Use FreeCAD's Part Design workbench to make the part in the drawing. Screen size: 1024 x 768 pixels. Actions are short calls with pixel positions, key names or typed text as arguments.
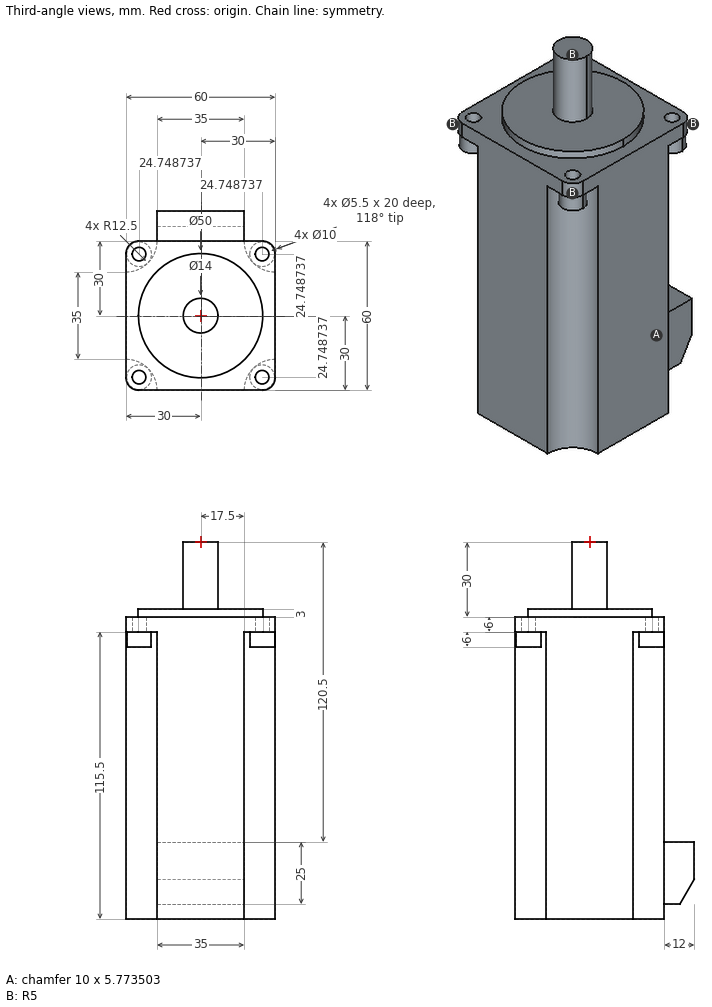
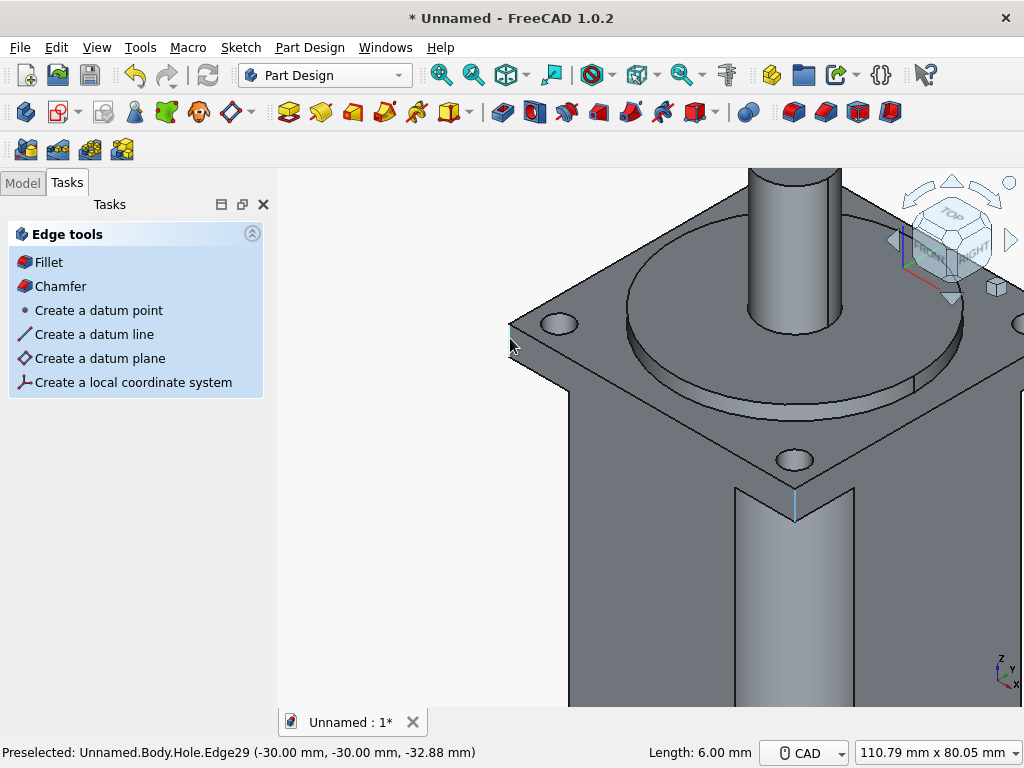
click(442, 76)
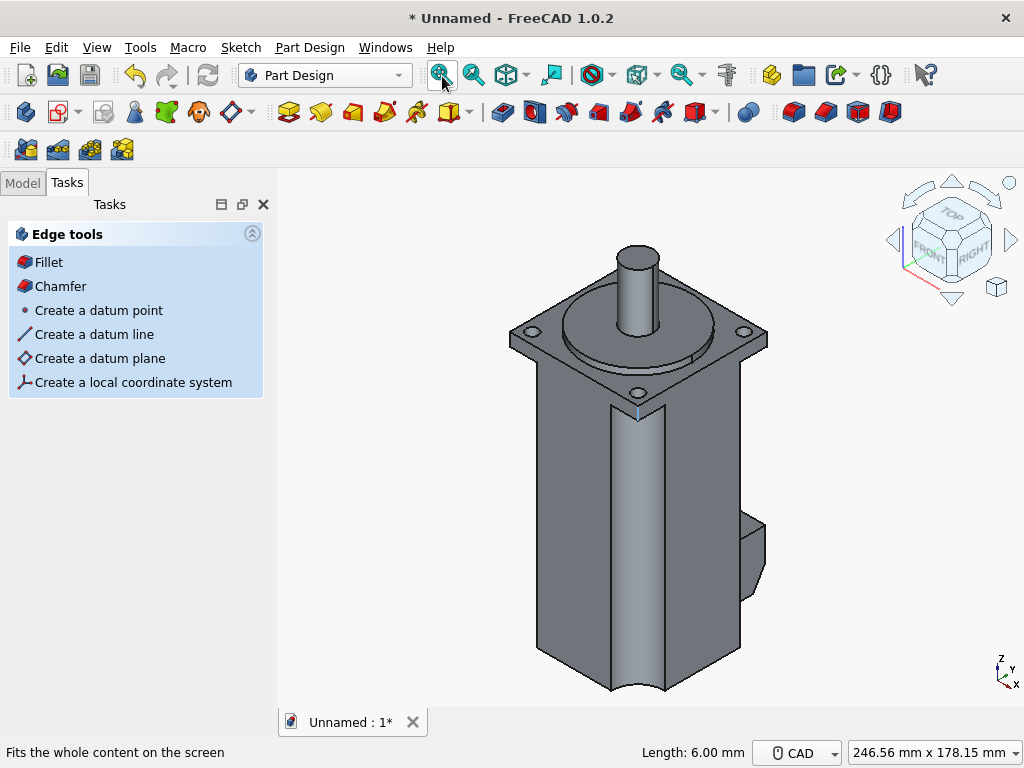
key(2)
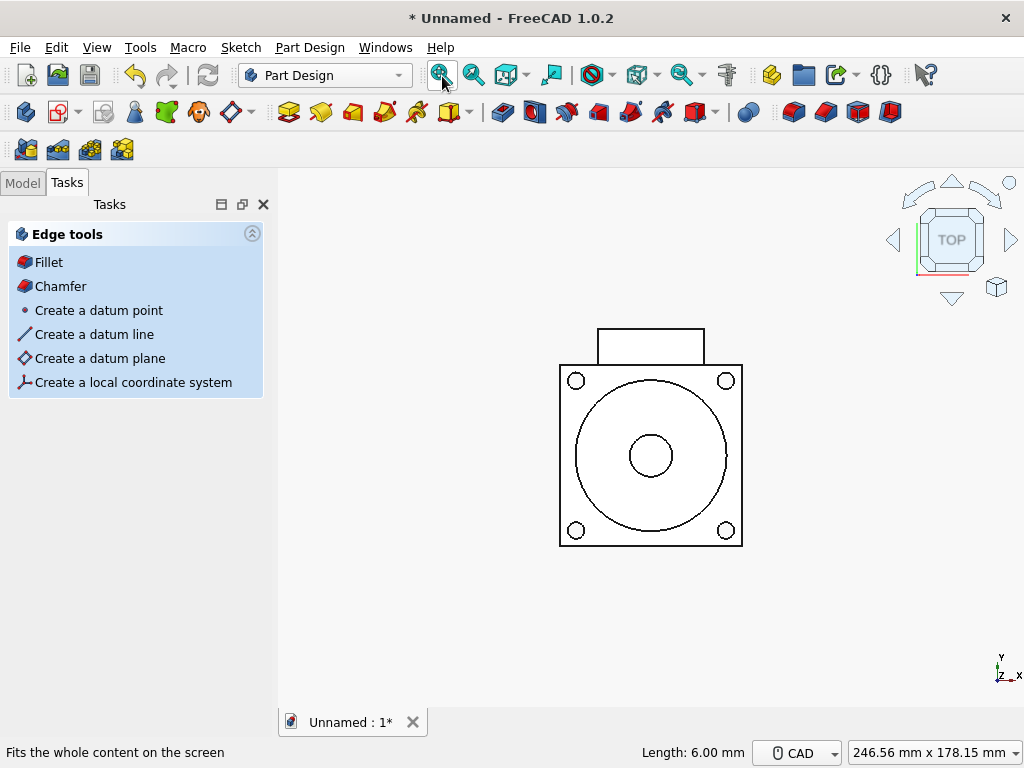
click(442, 76)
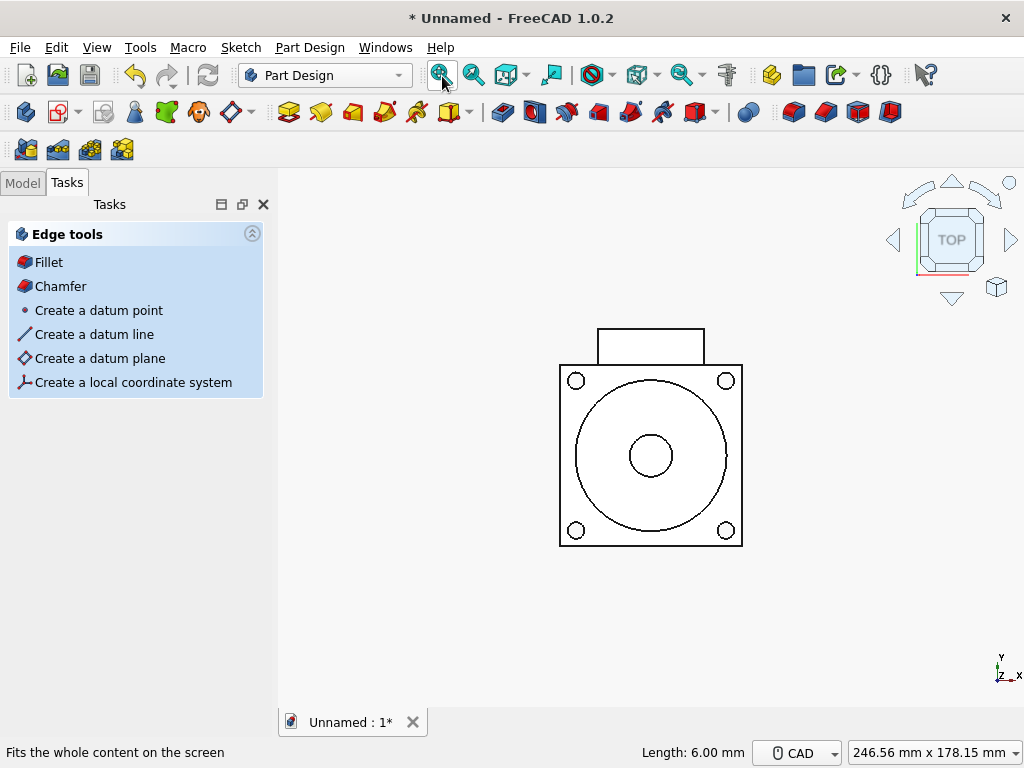
scroll(560, 545, up, 4)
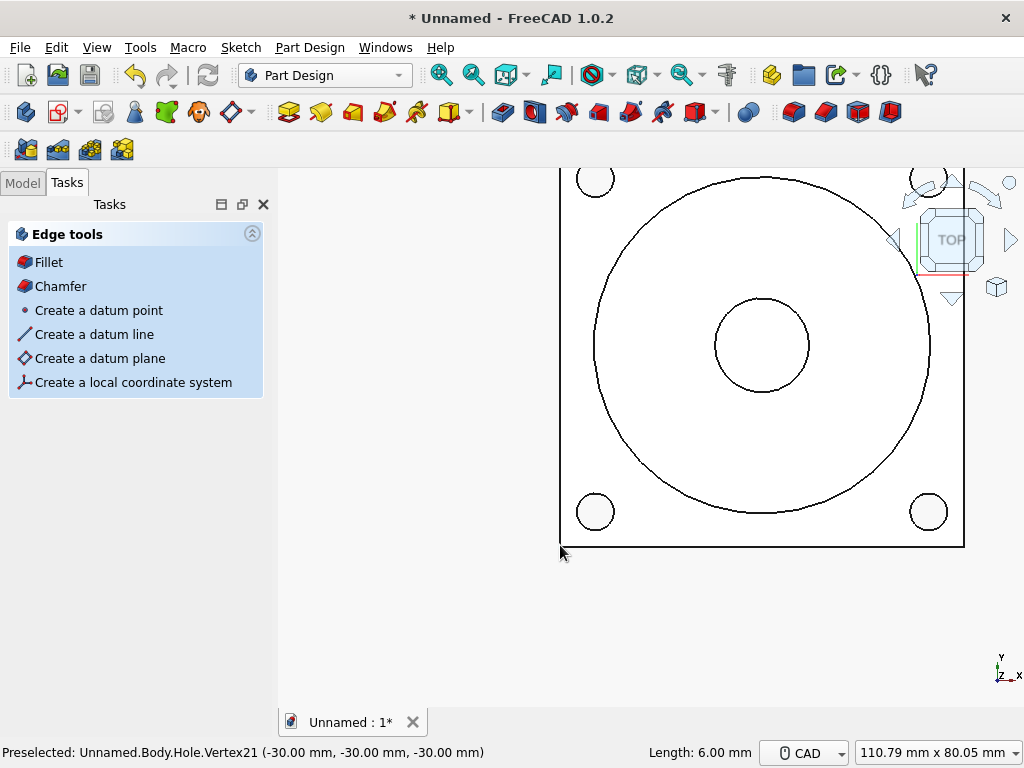
click(442, 76)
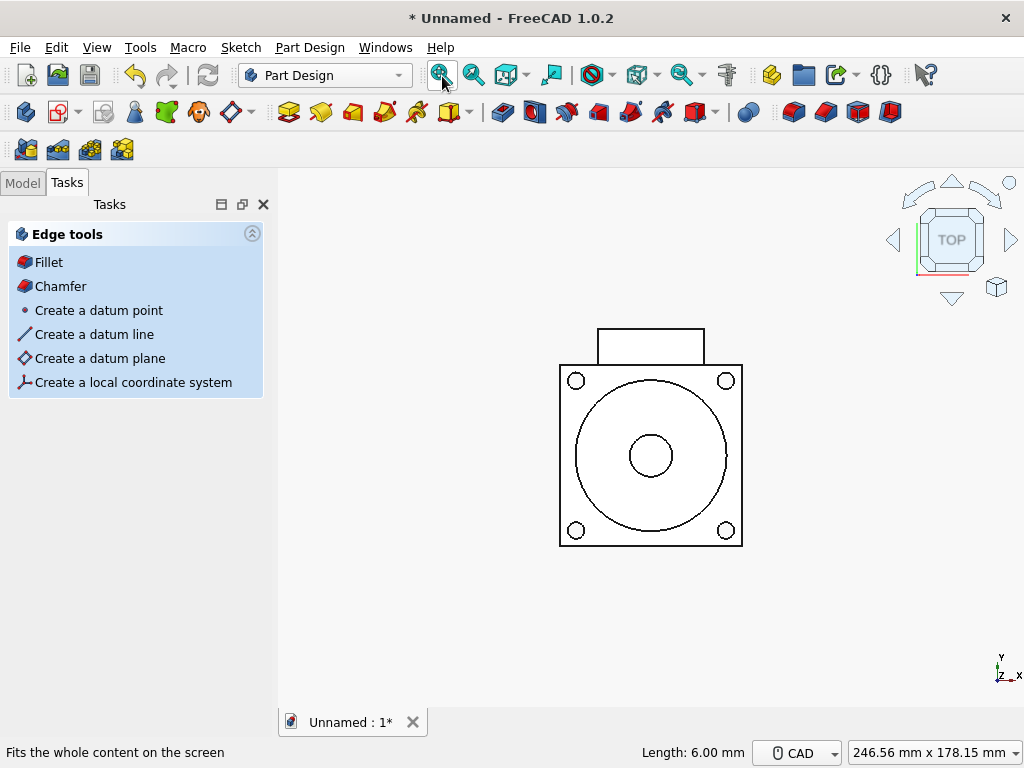
key(0)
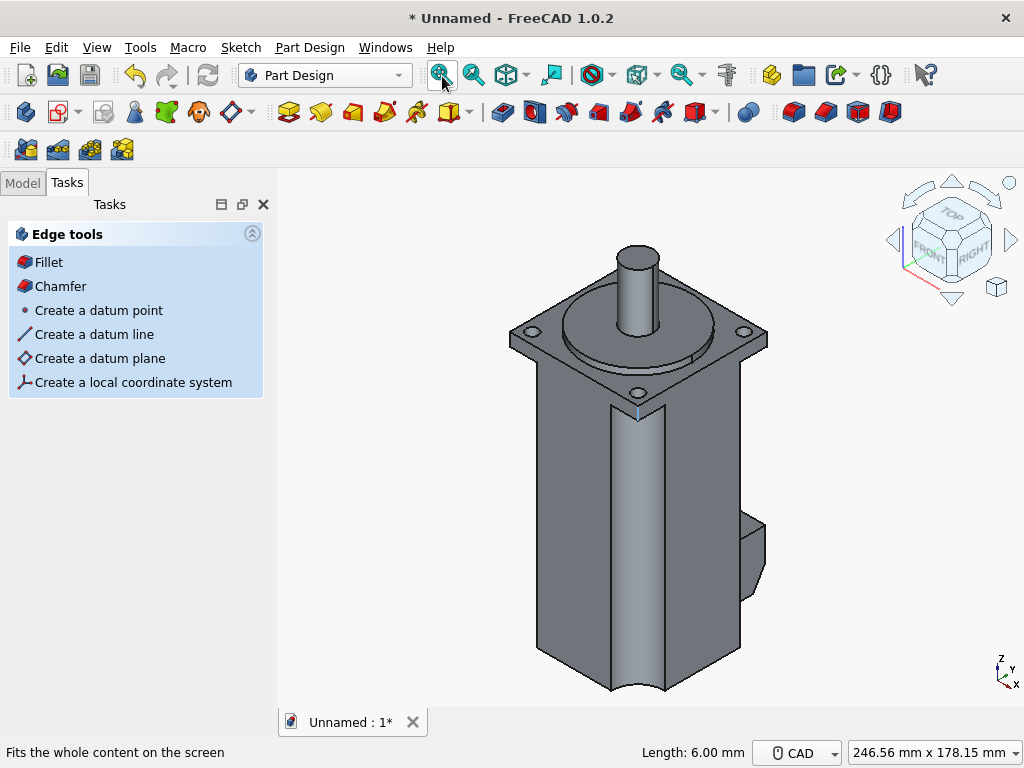
scroll(510, 338, up, 4)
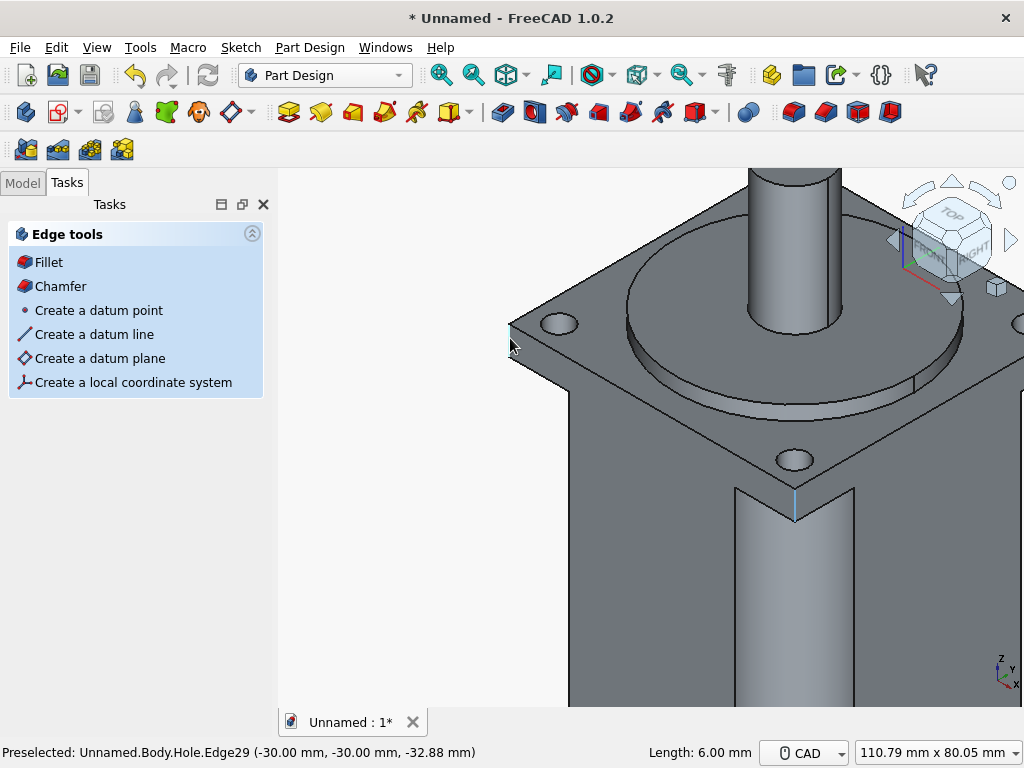
click(442, 76)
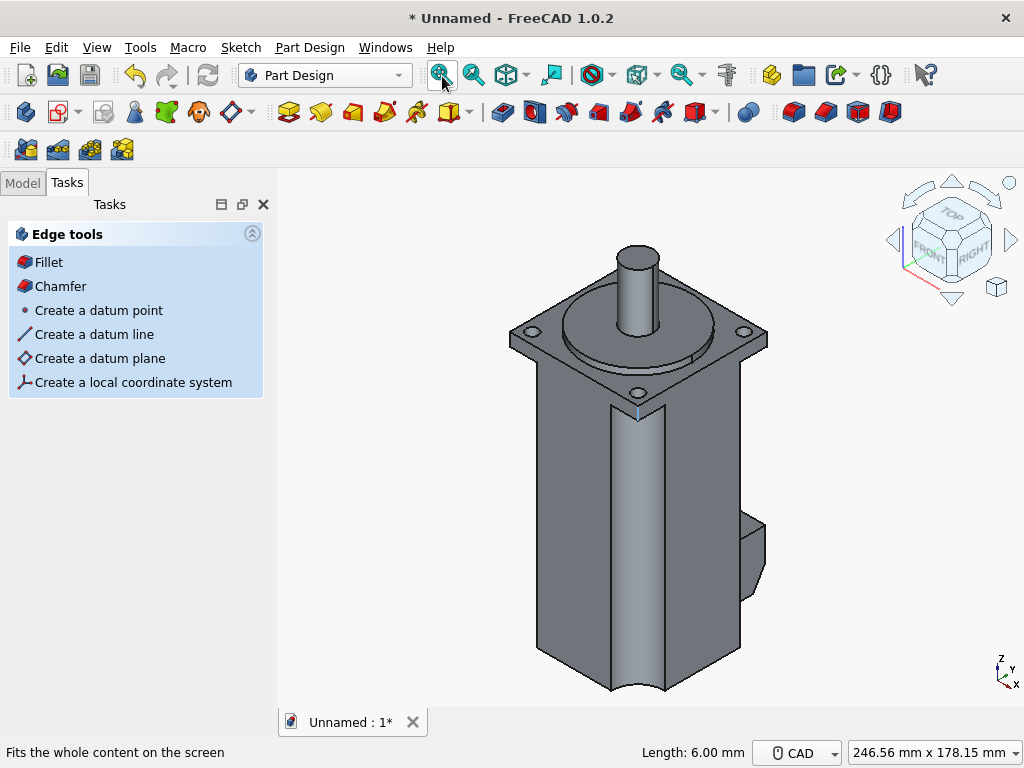
key(1)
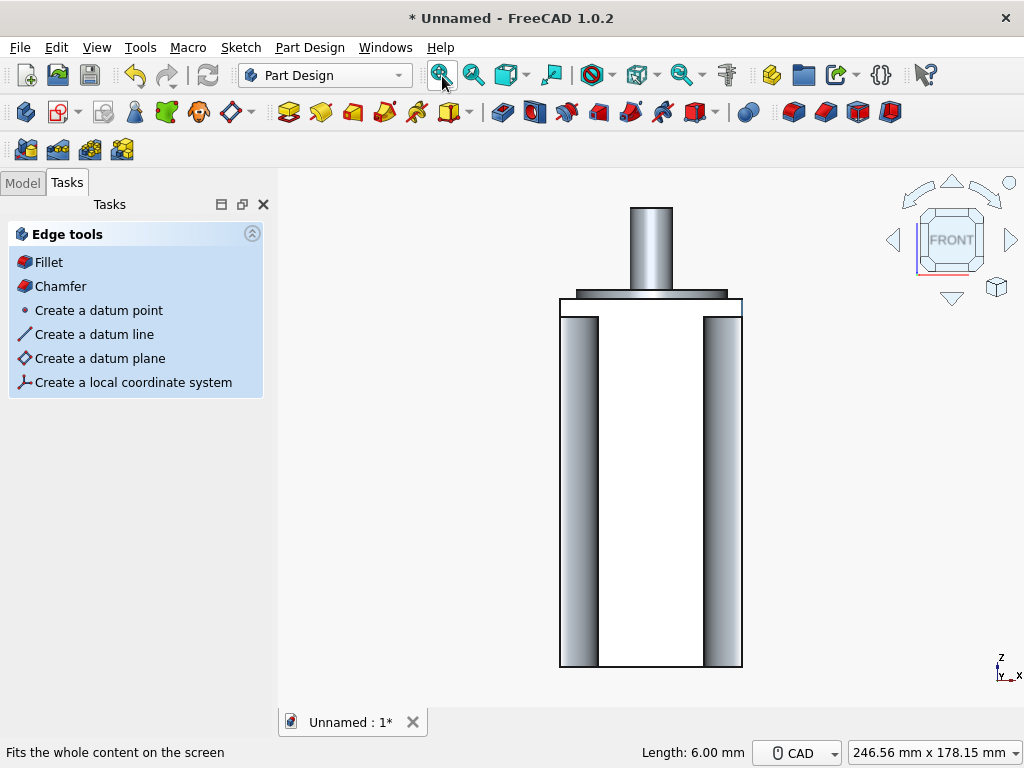
click(560, 307, ctrl)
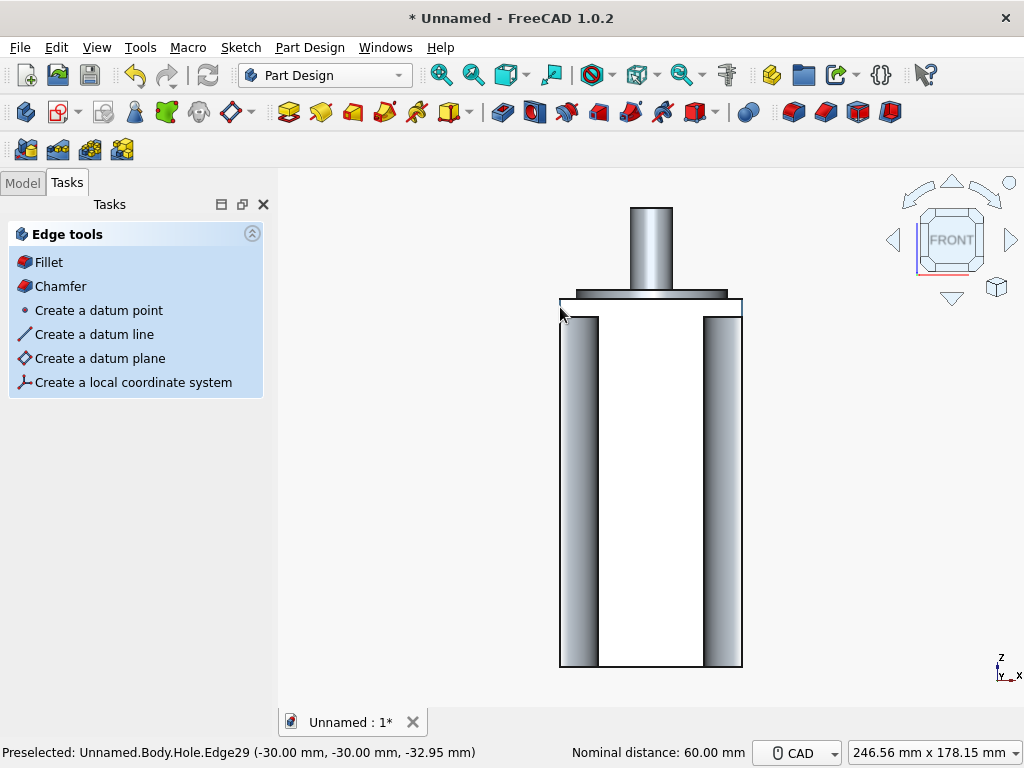
scroll(560, 307, up, 4)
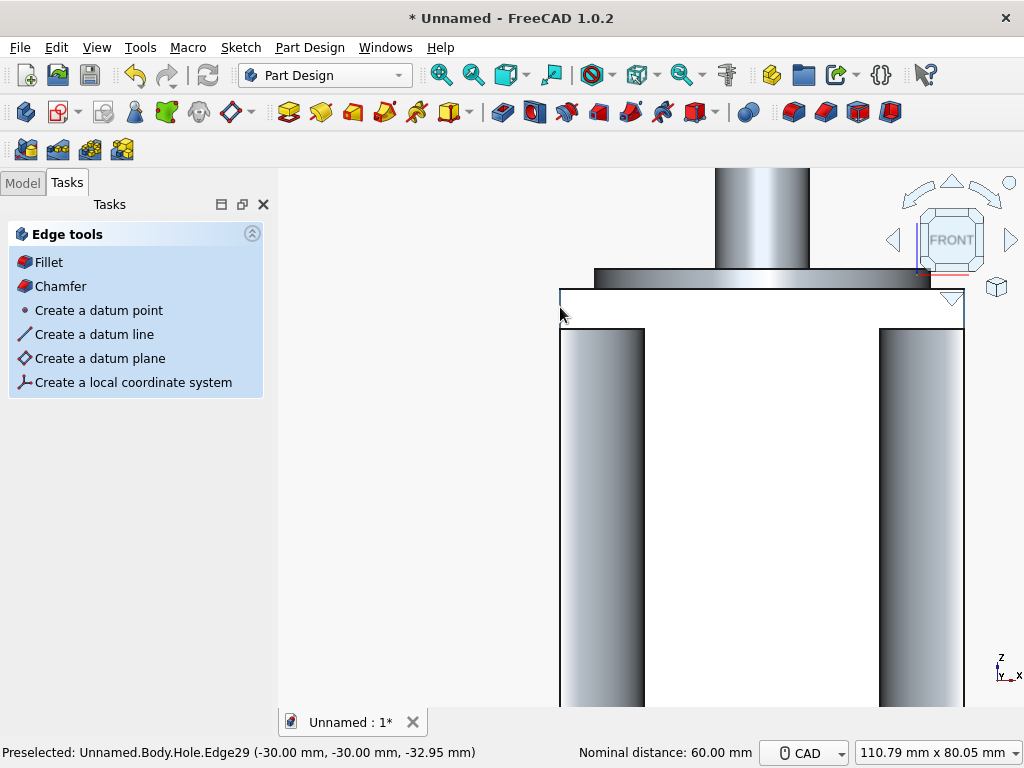
click(442, 76)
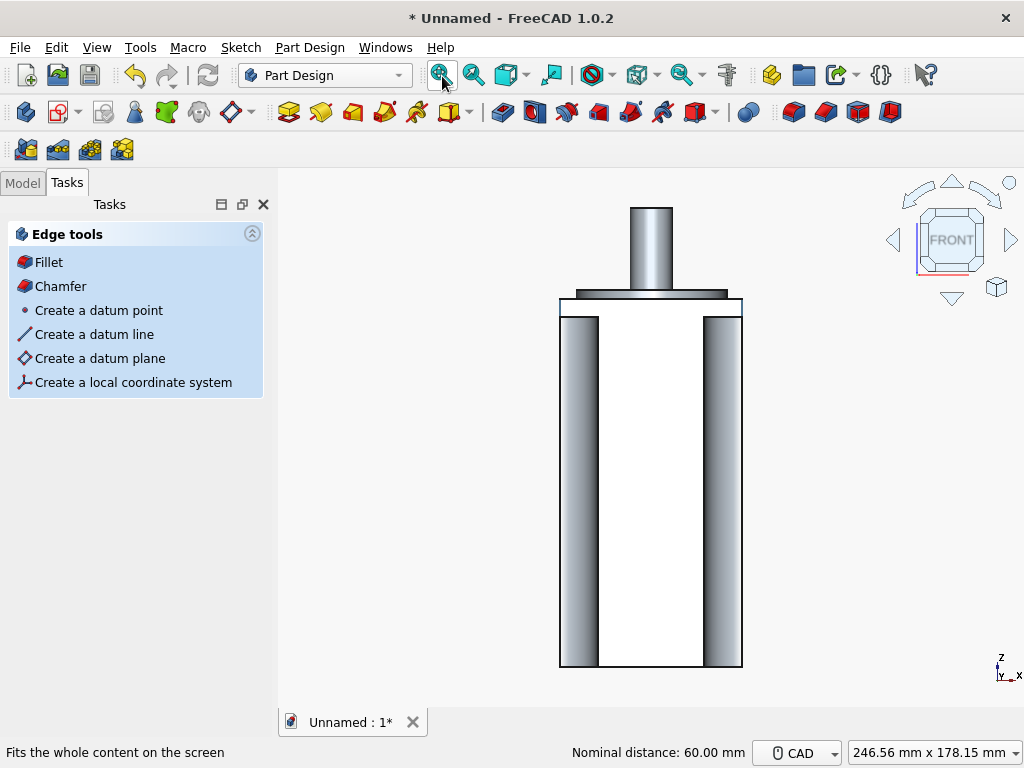
key(3)